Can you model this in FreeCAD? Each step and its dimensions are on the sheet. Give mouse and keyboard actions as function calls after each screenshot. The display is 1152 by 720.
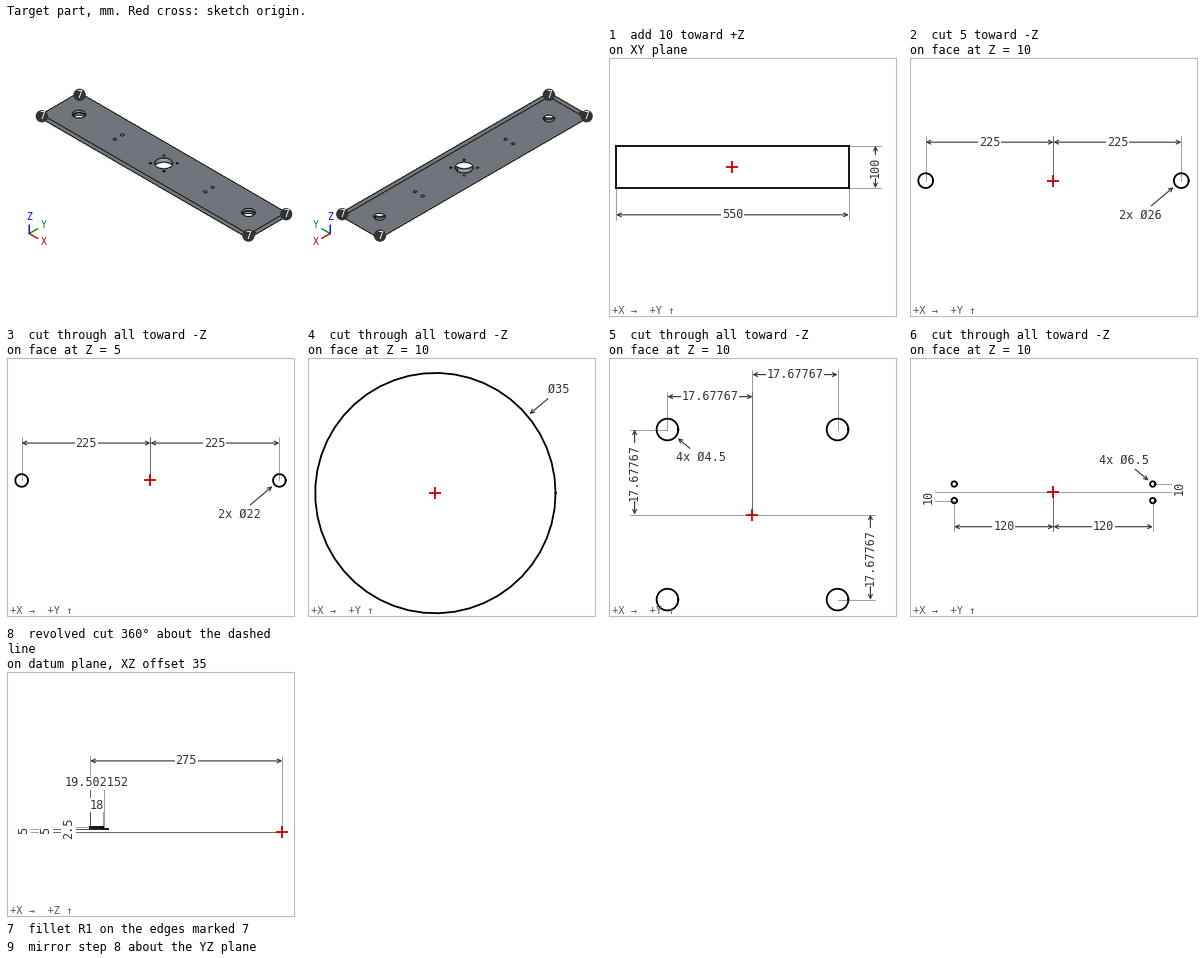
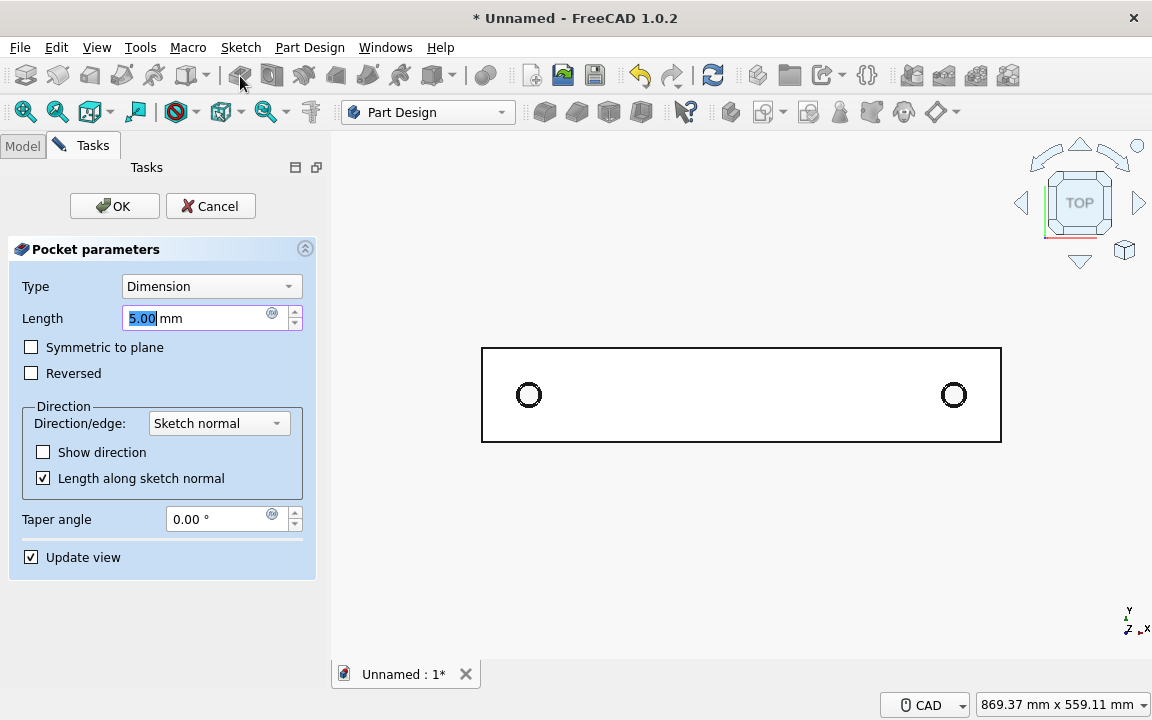
click(212, 286)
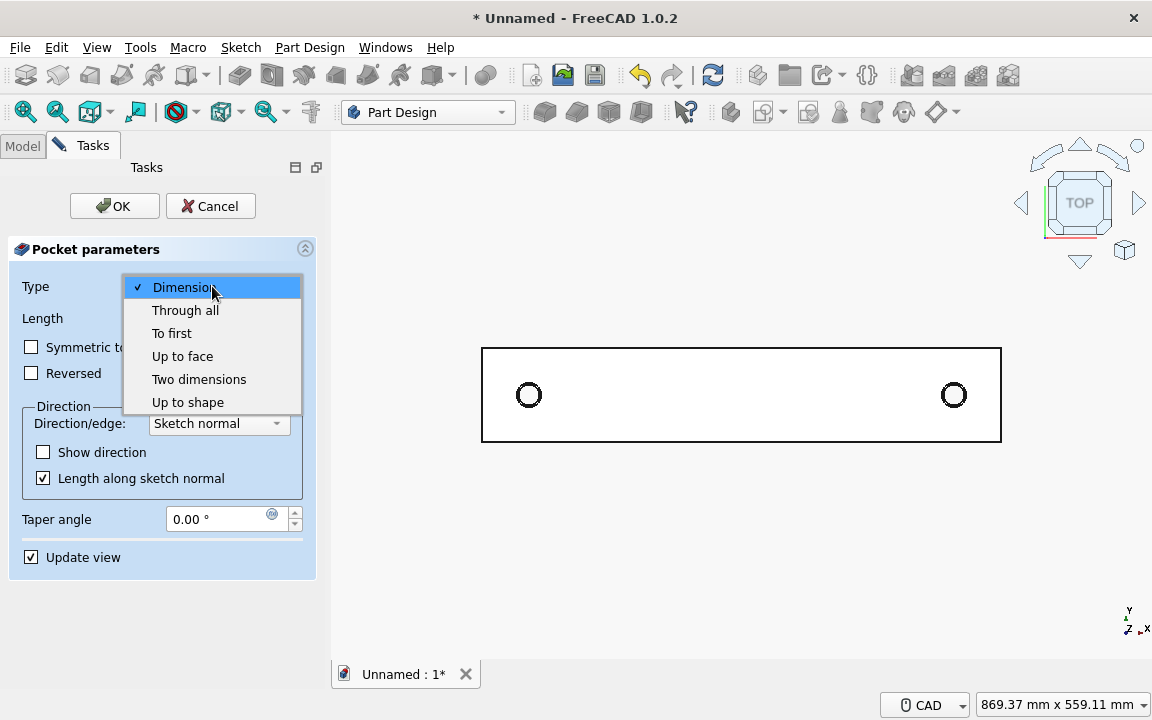
click(212, 310)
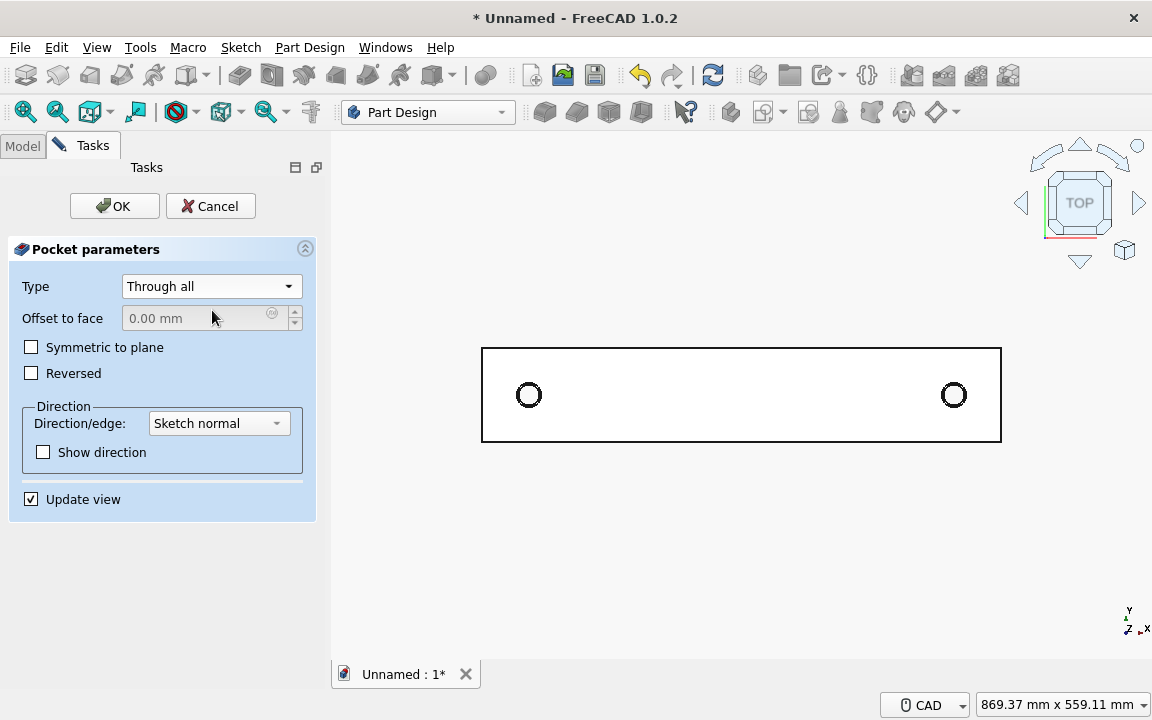
click(115, 206)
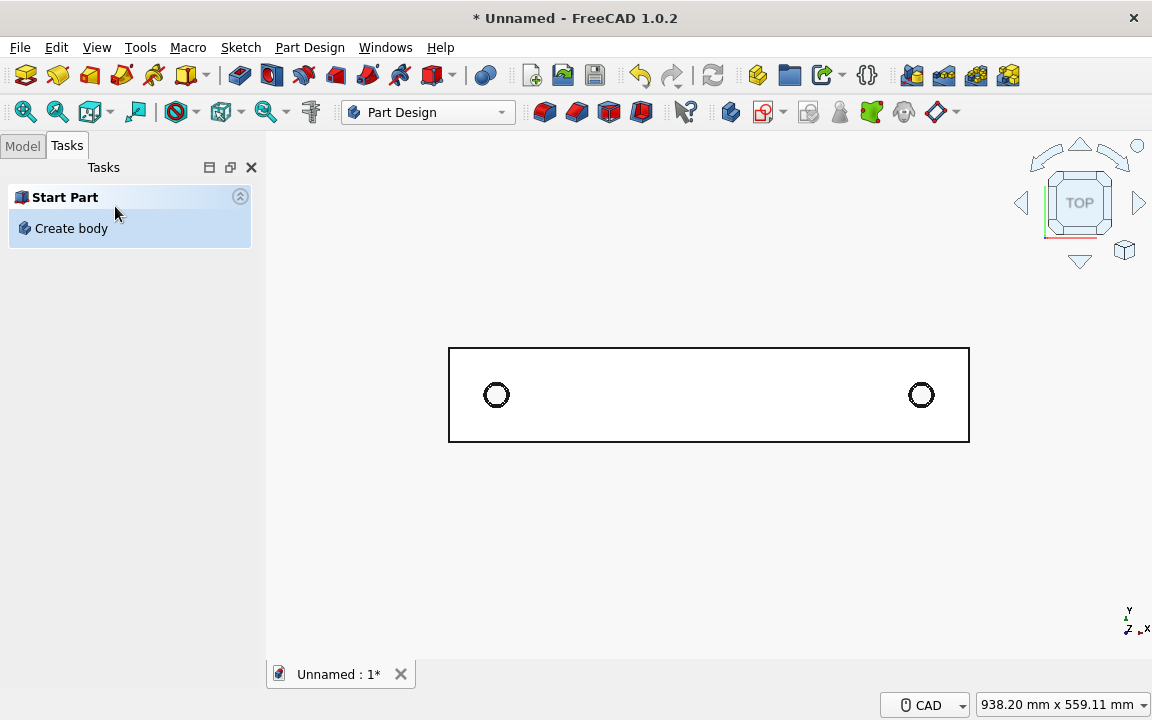
click(857, 394)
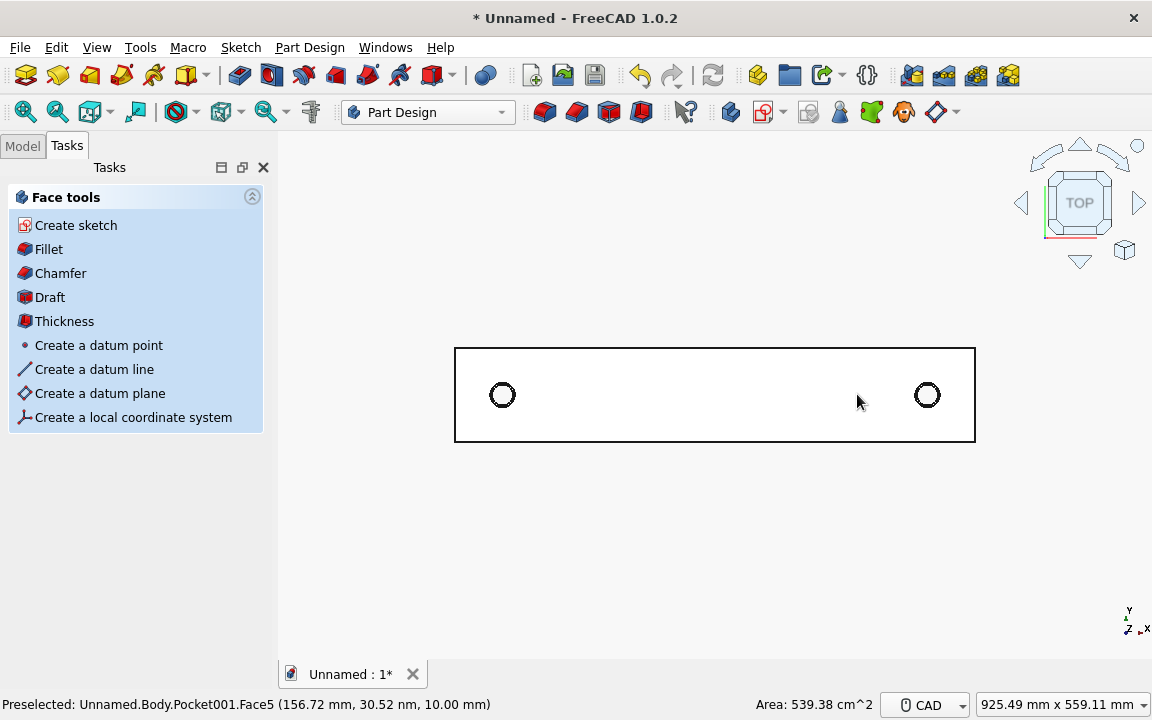
click(764, 112)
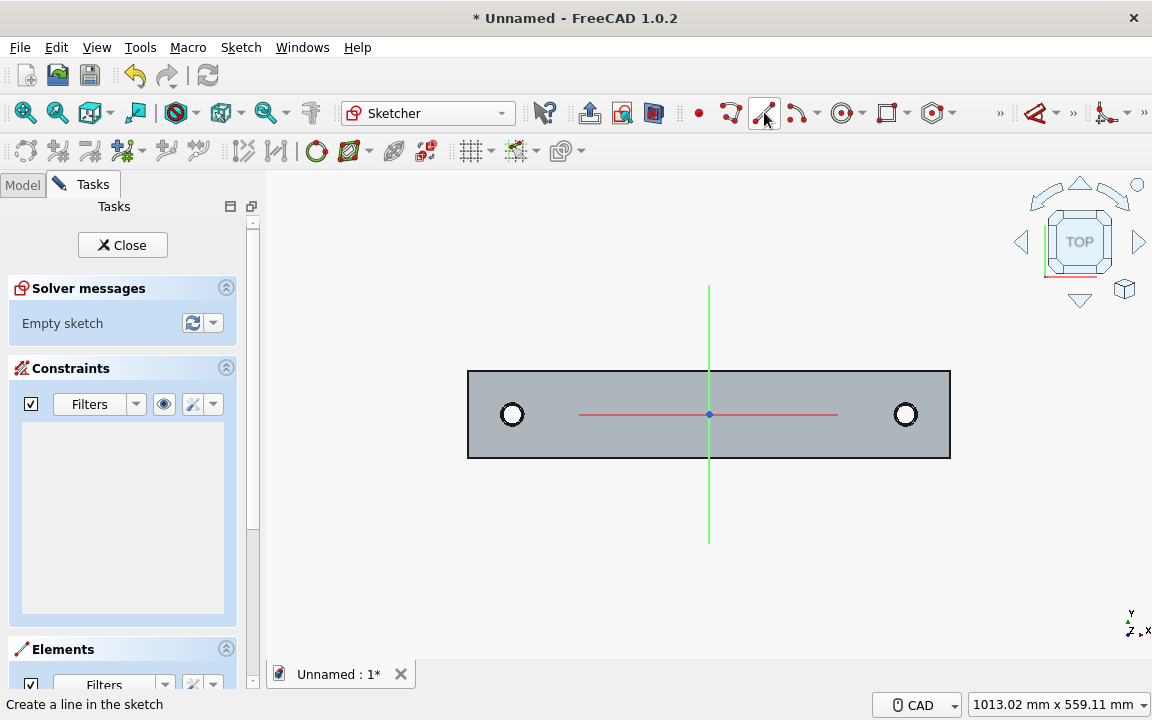
scroll(716, 415, up, 12)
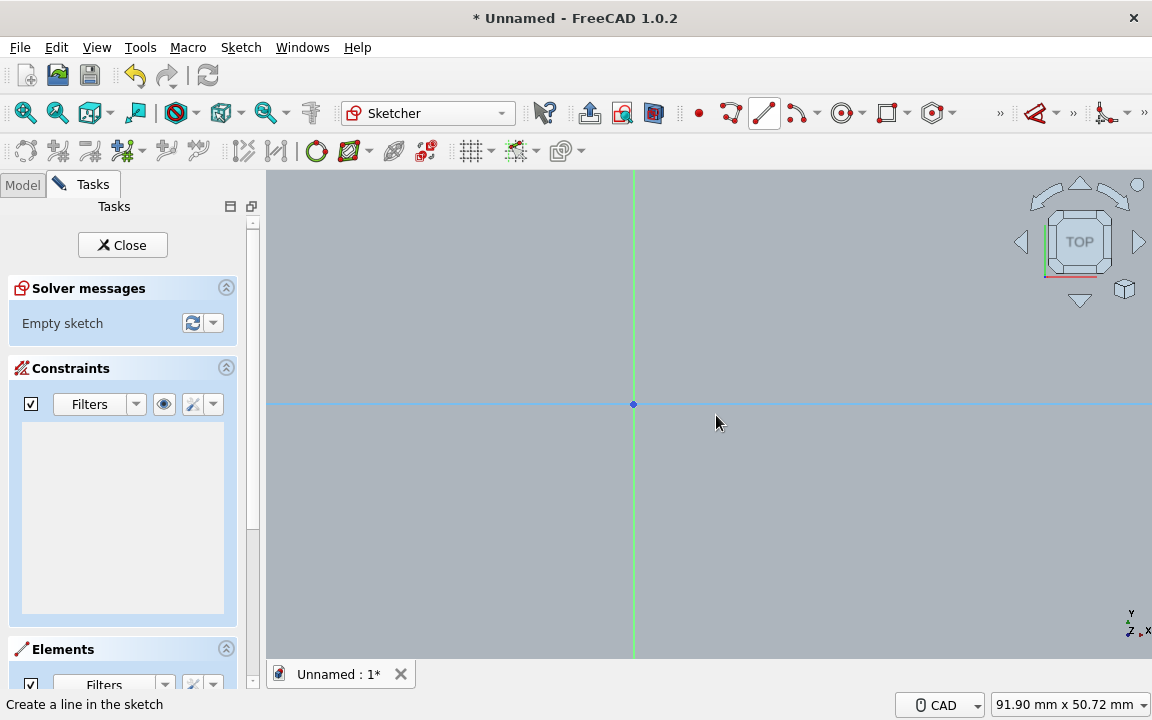
click(842, 114)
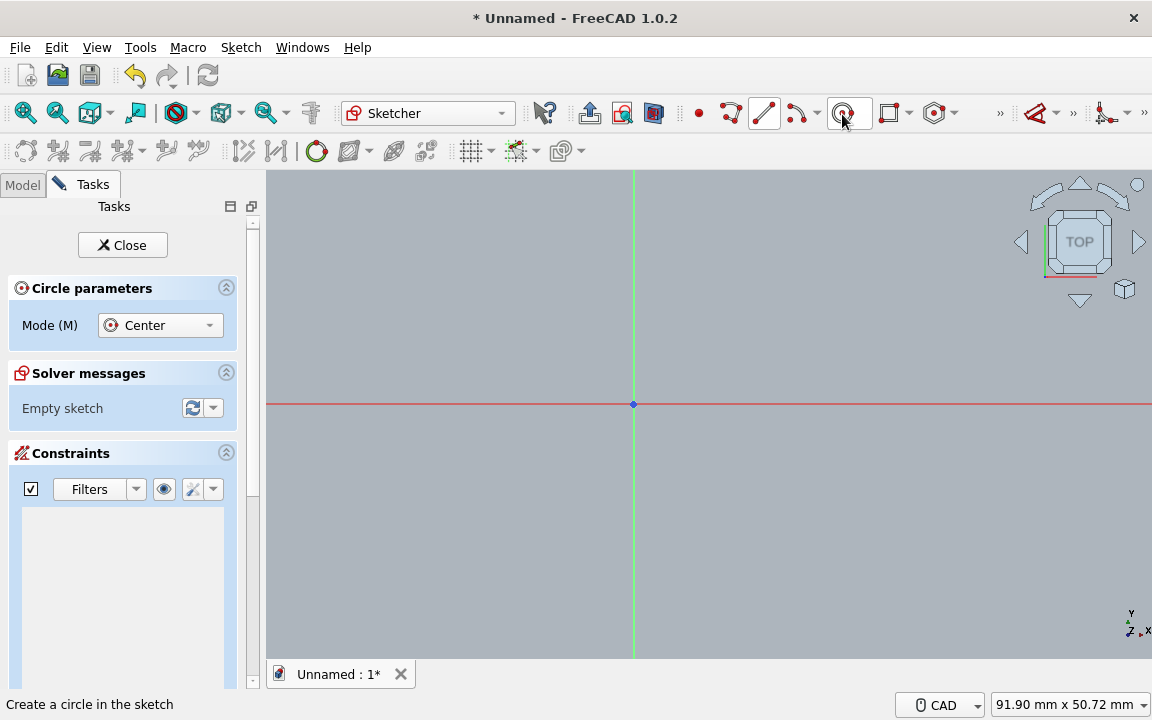
click(634, 404)
move(753, 285)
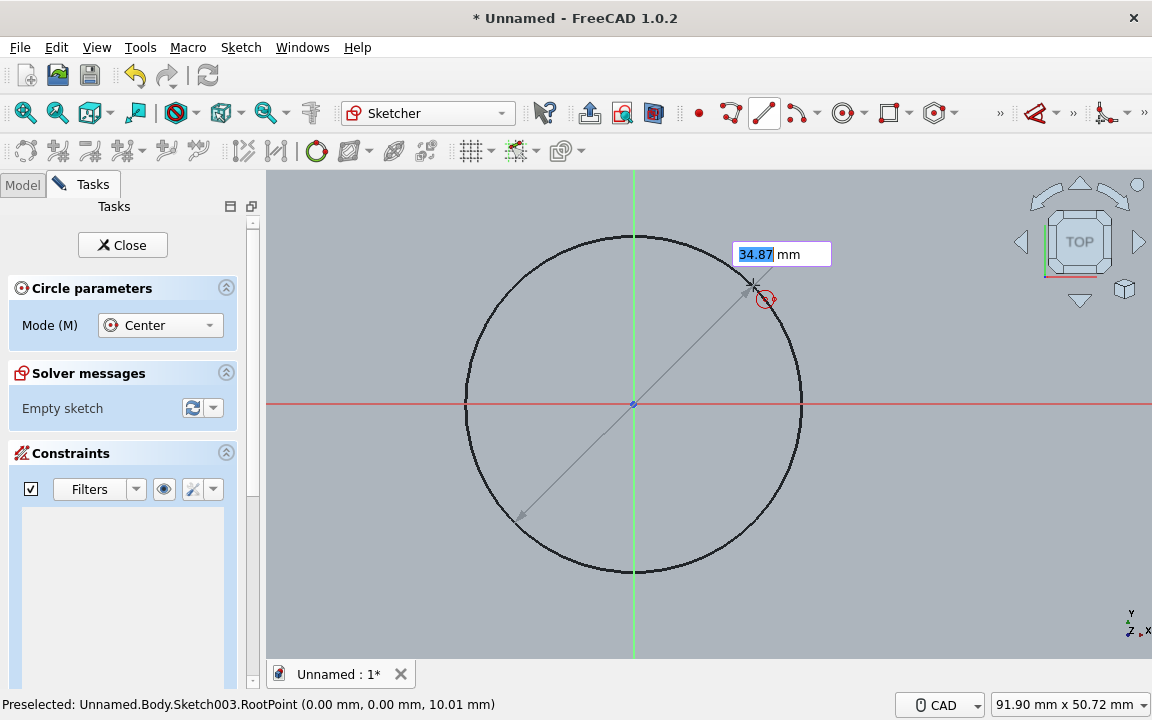
text(35)
key(Return)
key(Escape)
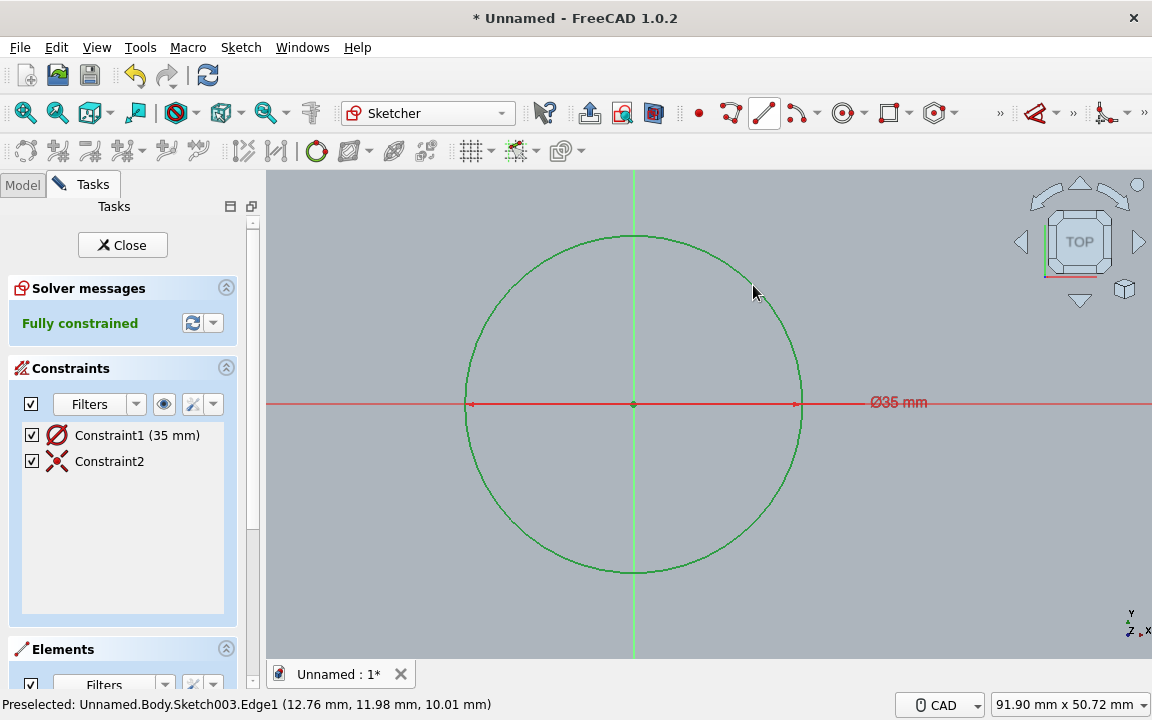
click(123, 245)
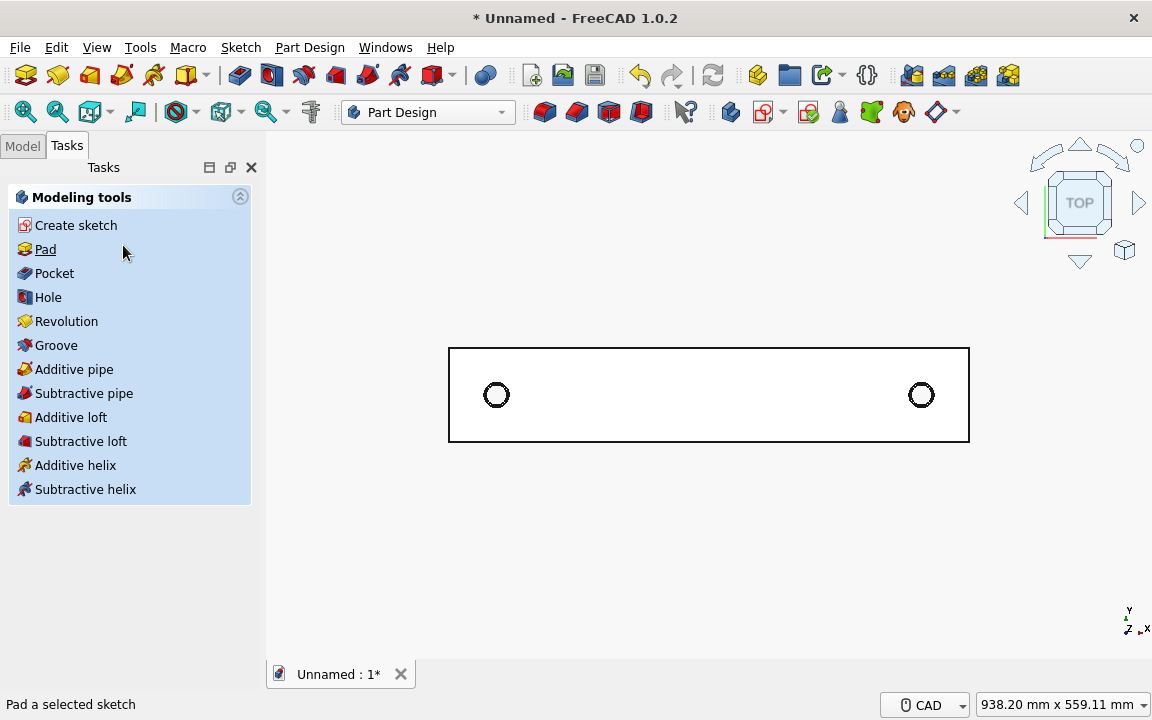
click(240, 76)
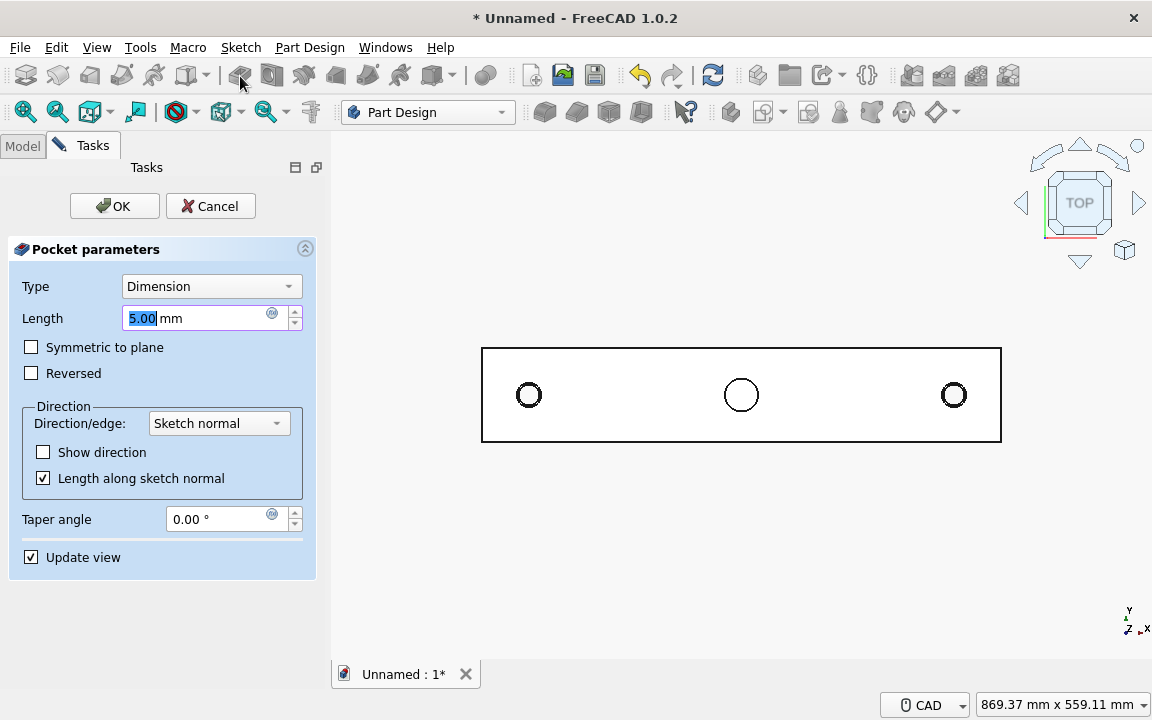
click(212, 286)